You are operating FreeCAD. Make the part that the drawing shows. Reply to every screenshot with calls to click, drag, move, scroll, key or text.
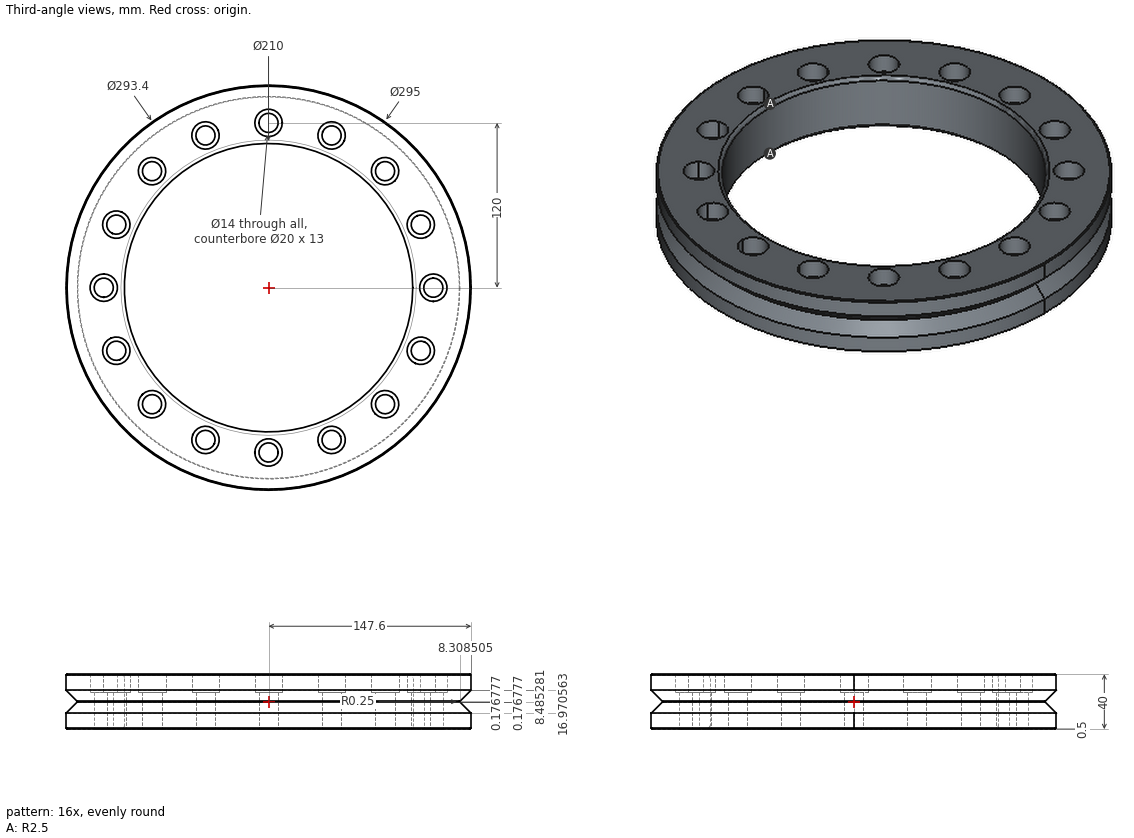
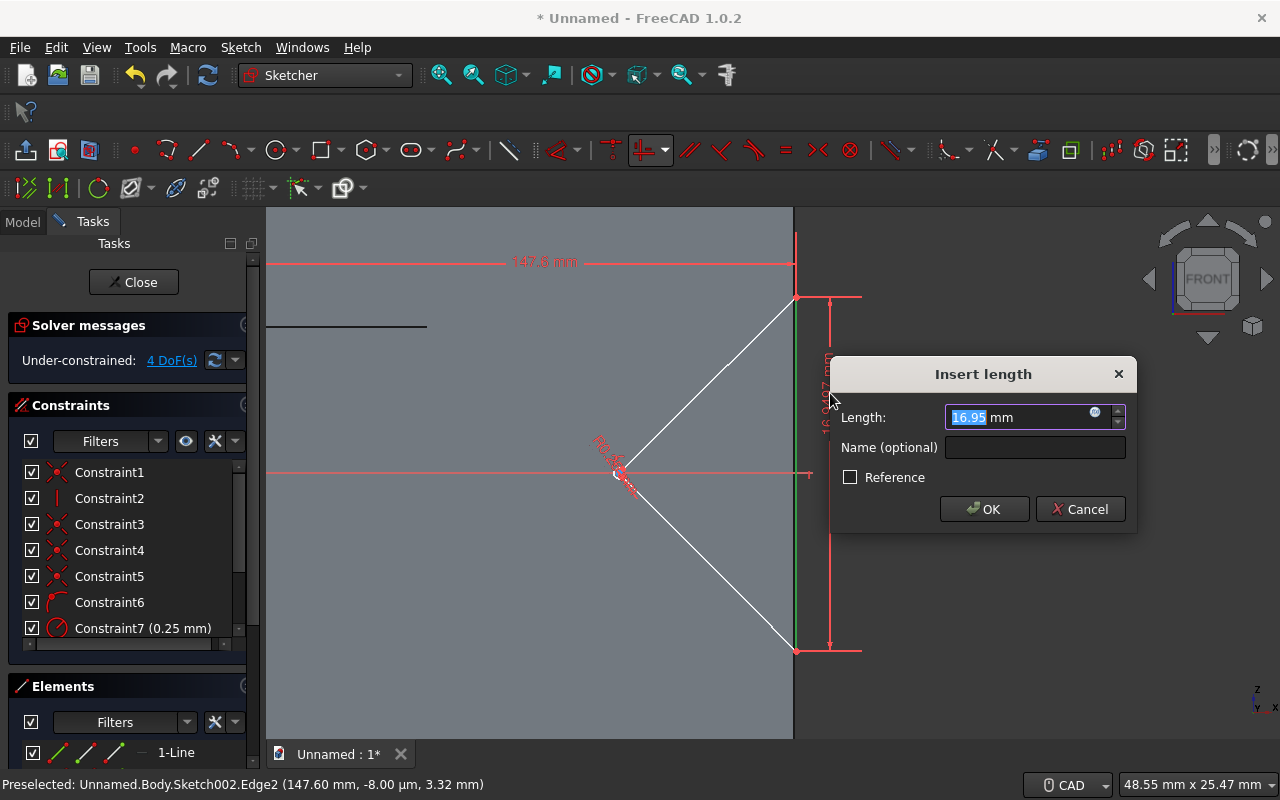
text(16.970563)
key(Return)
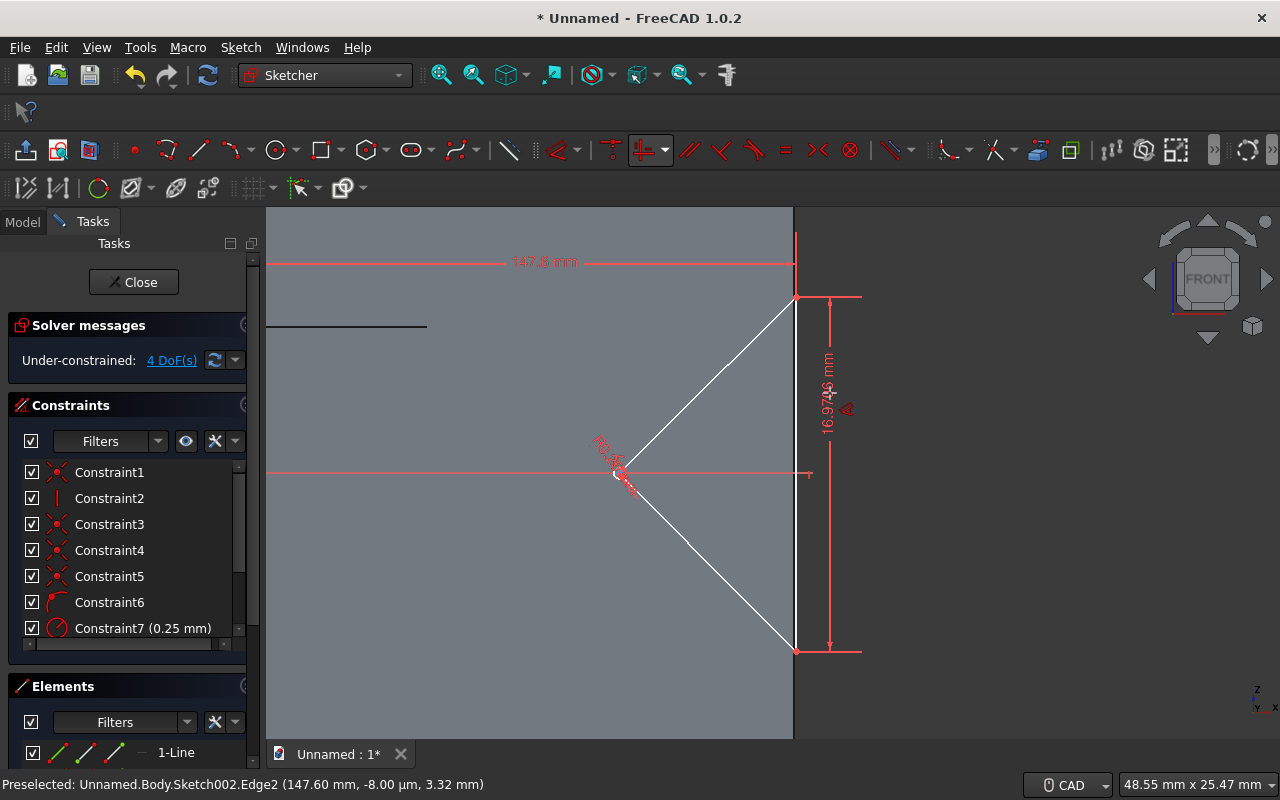
scroll(623, 470, up, 12)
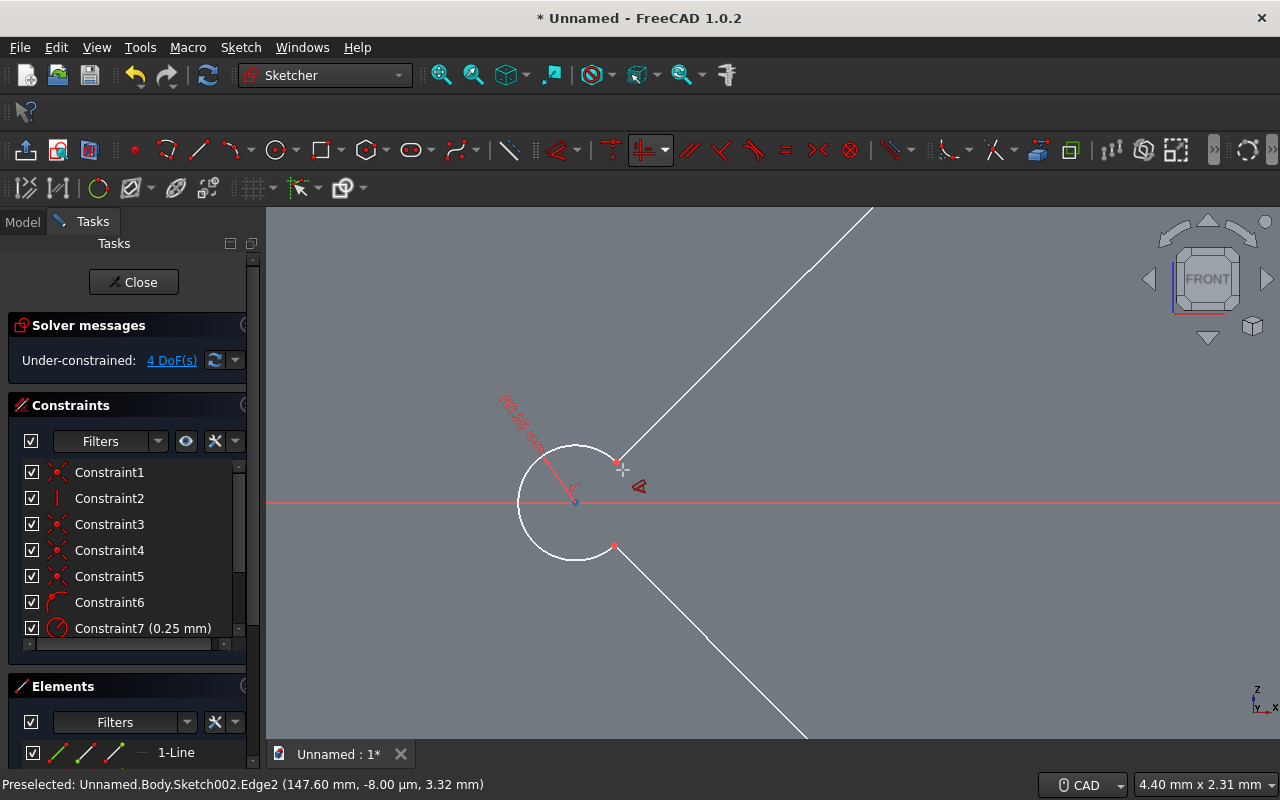
click(617, 462)
click(651, 483)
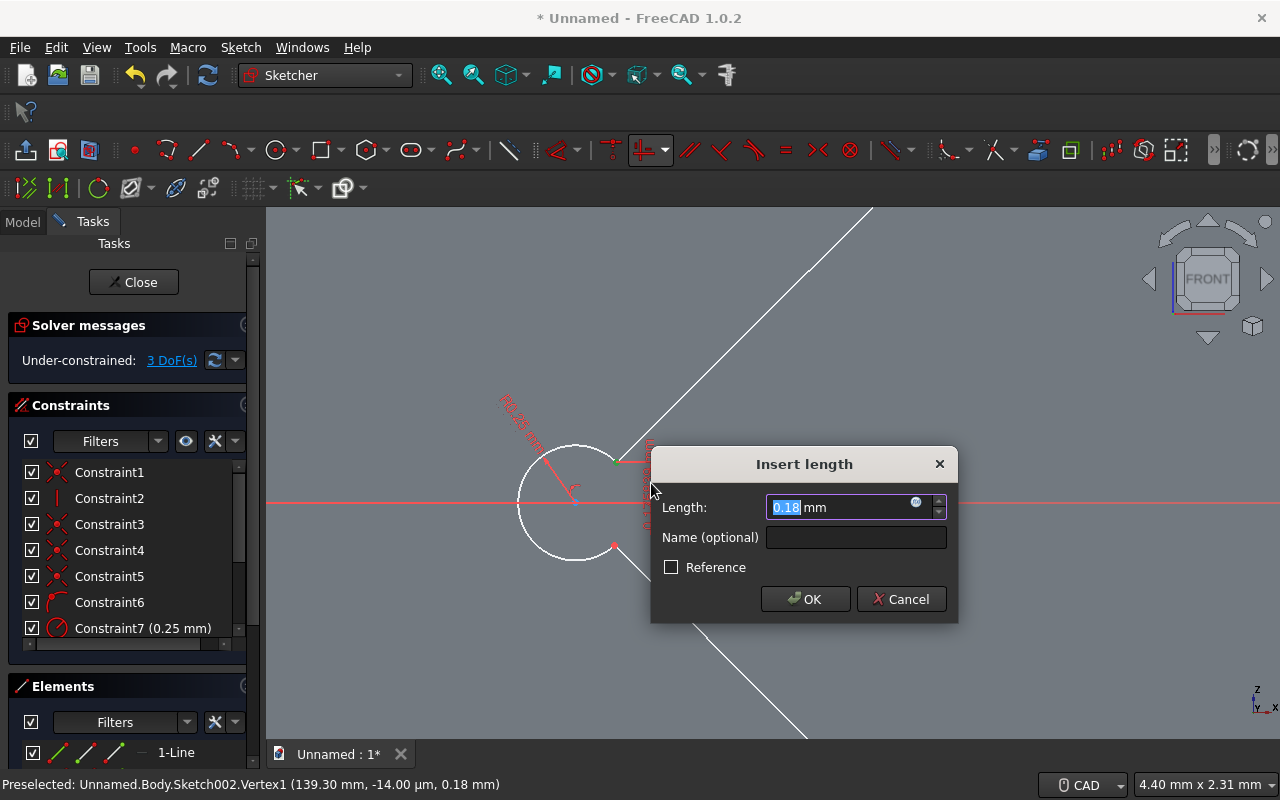
text(0.176777)
key(Return)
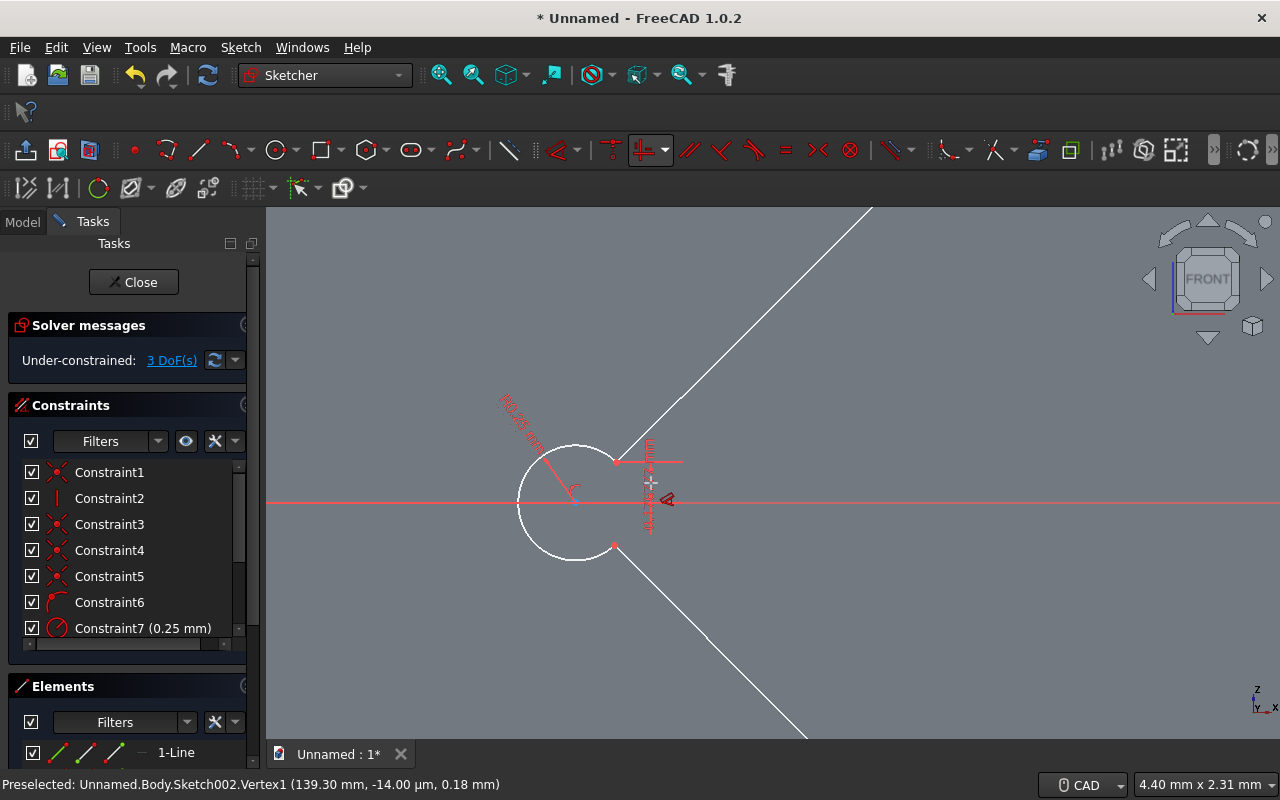
scroll(623, 470, down, 12)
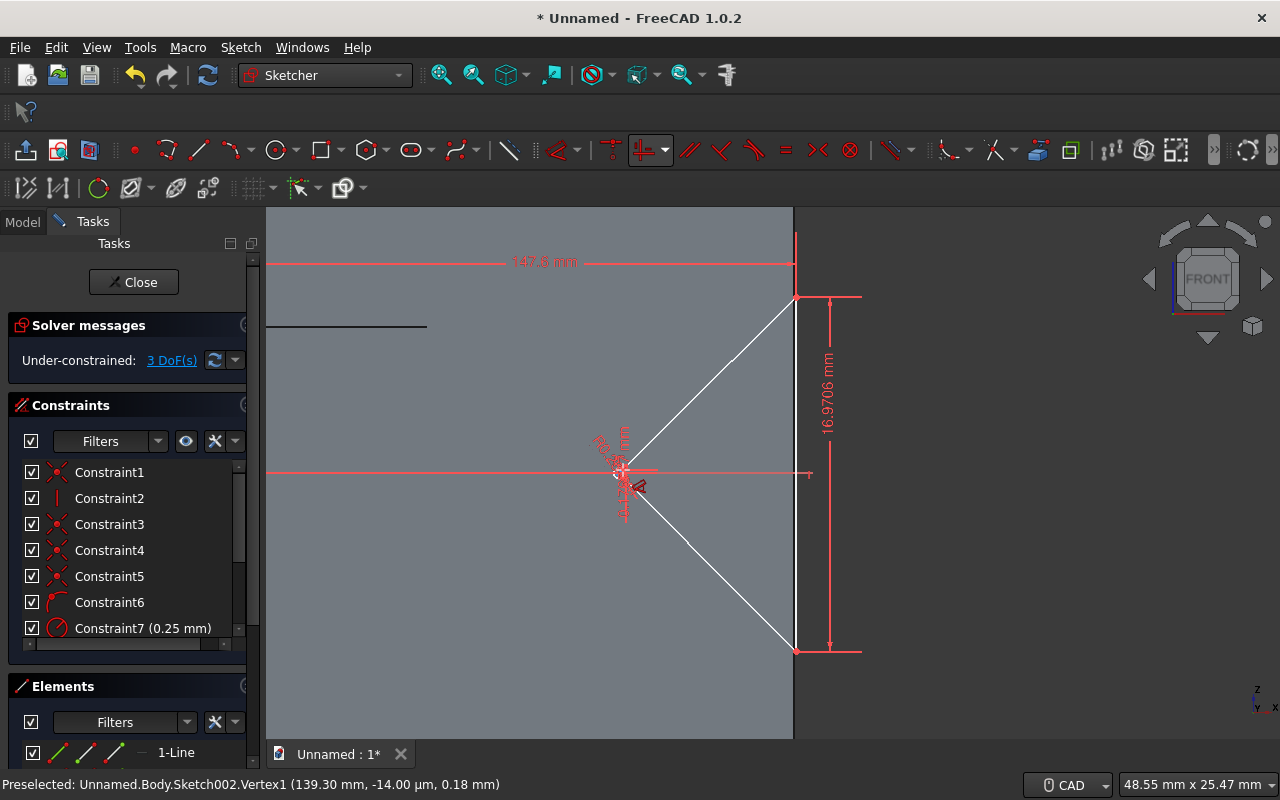
click(796, 297)
click(830, 345)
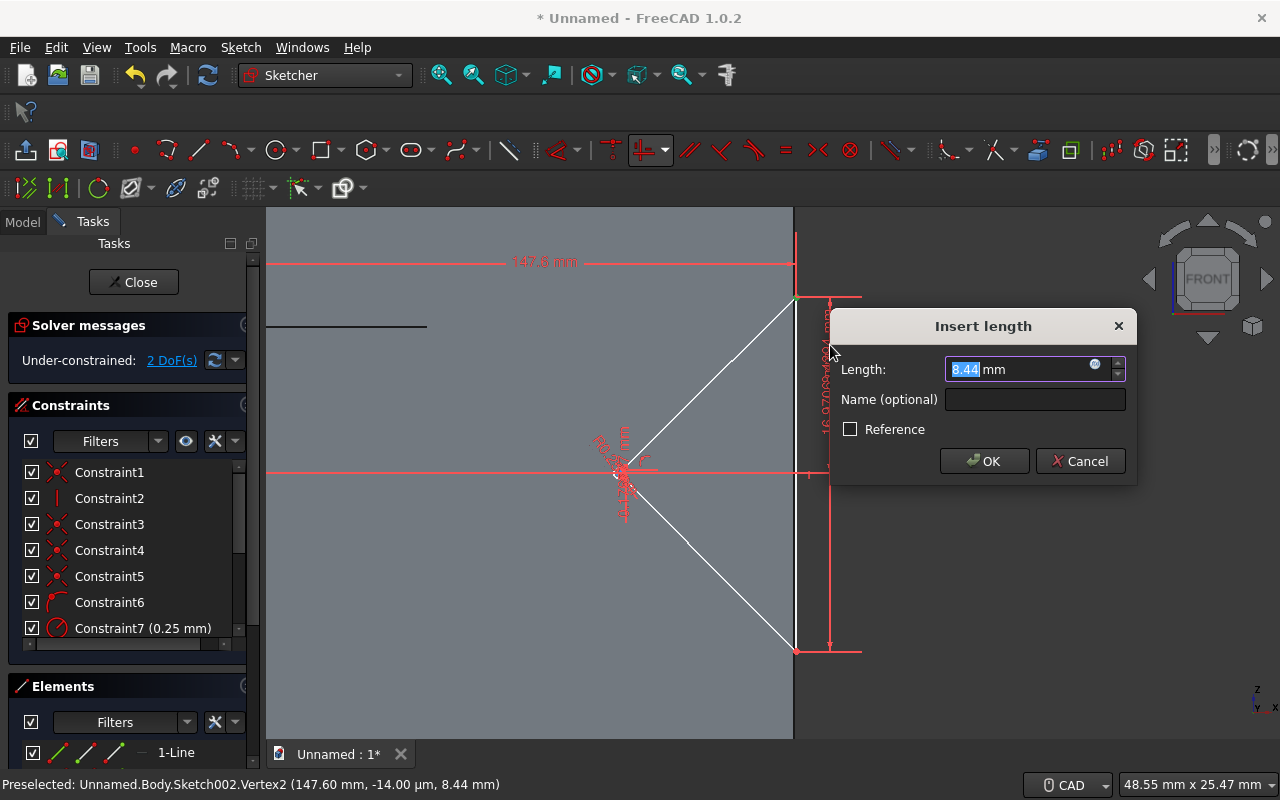
text(8.485281)
key(Return)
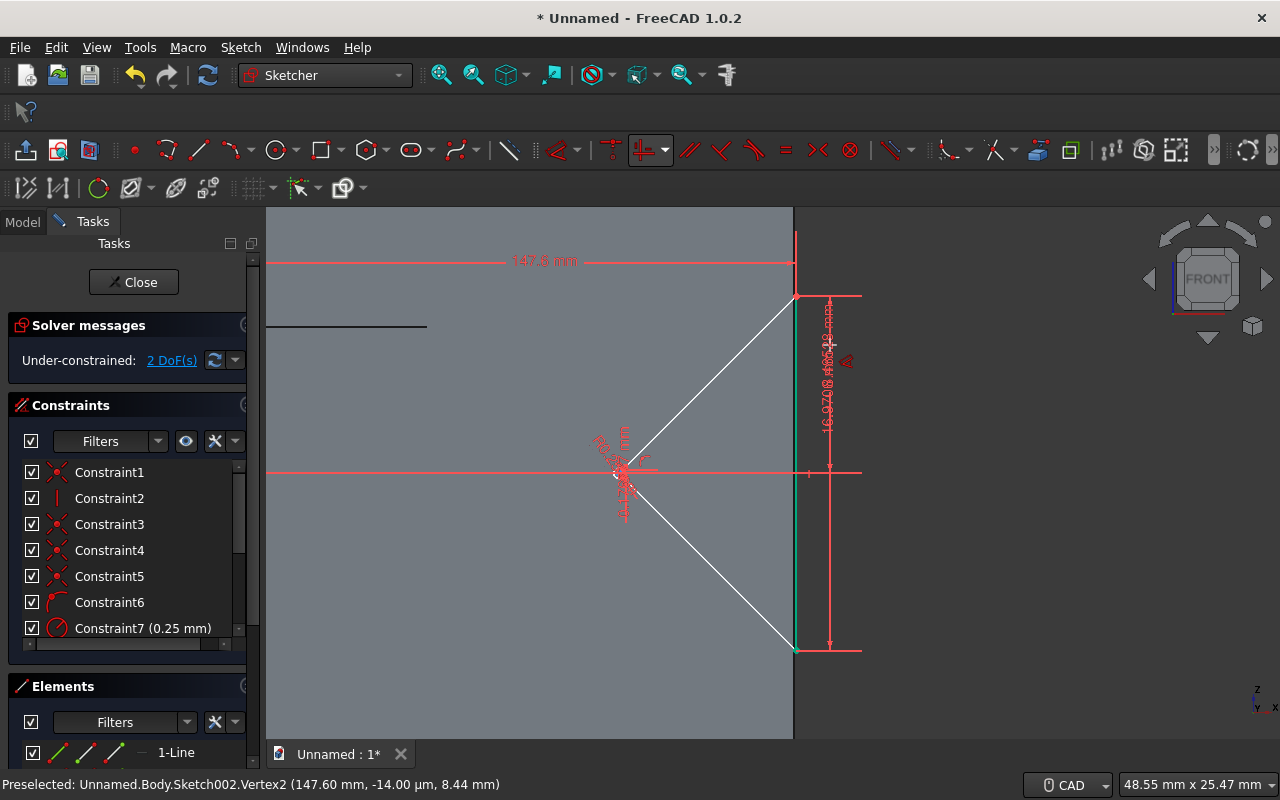
scroll(623, 477, up, 12)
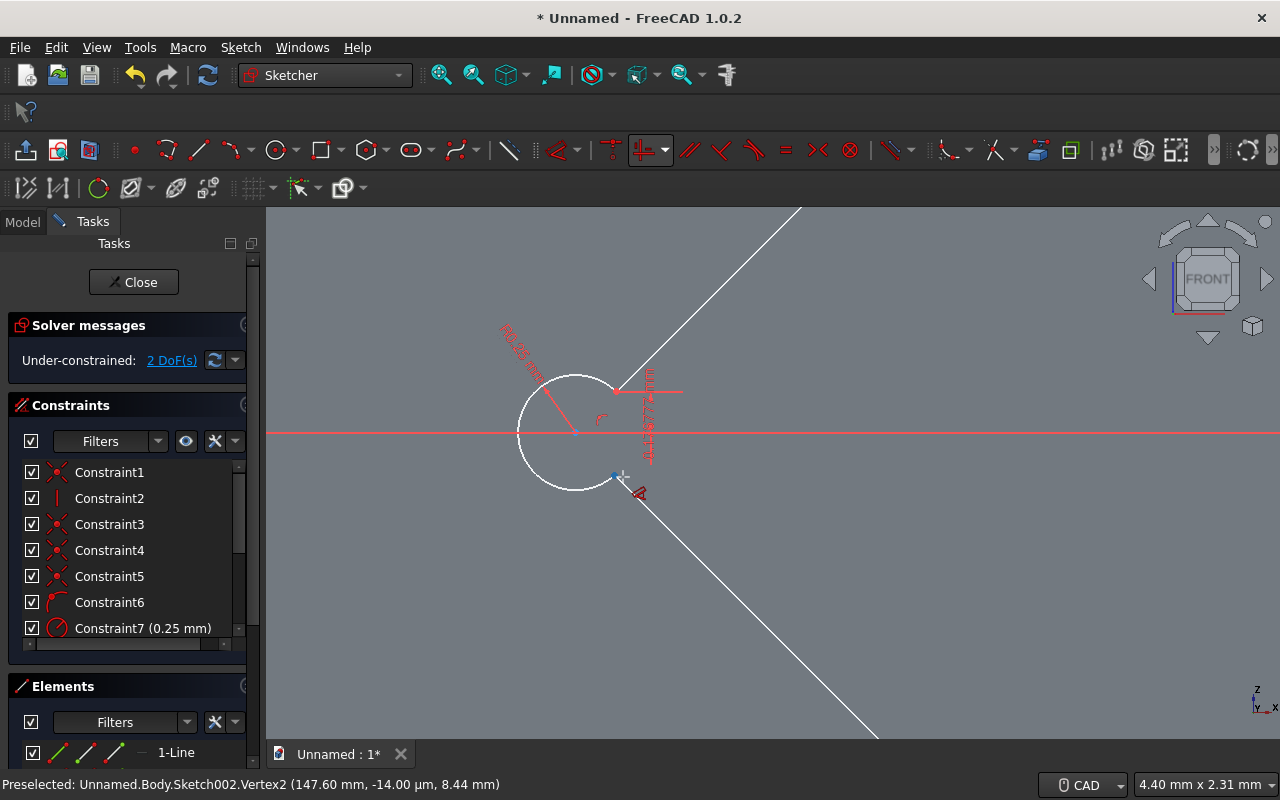
click(615, 475)
click(649, 454)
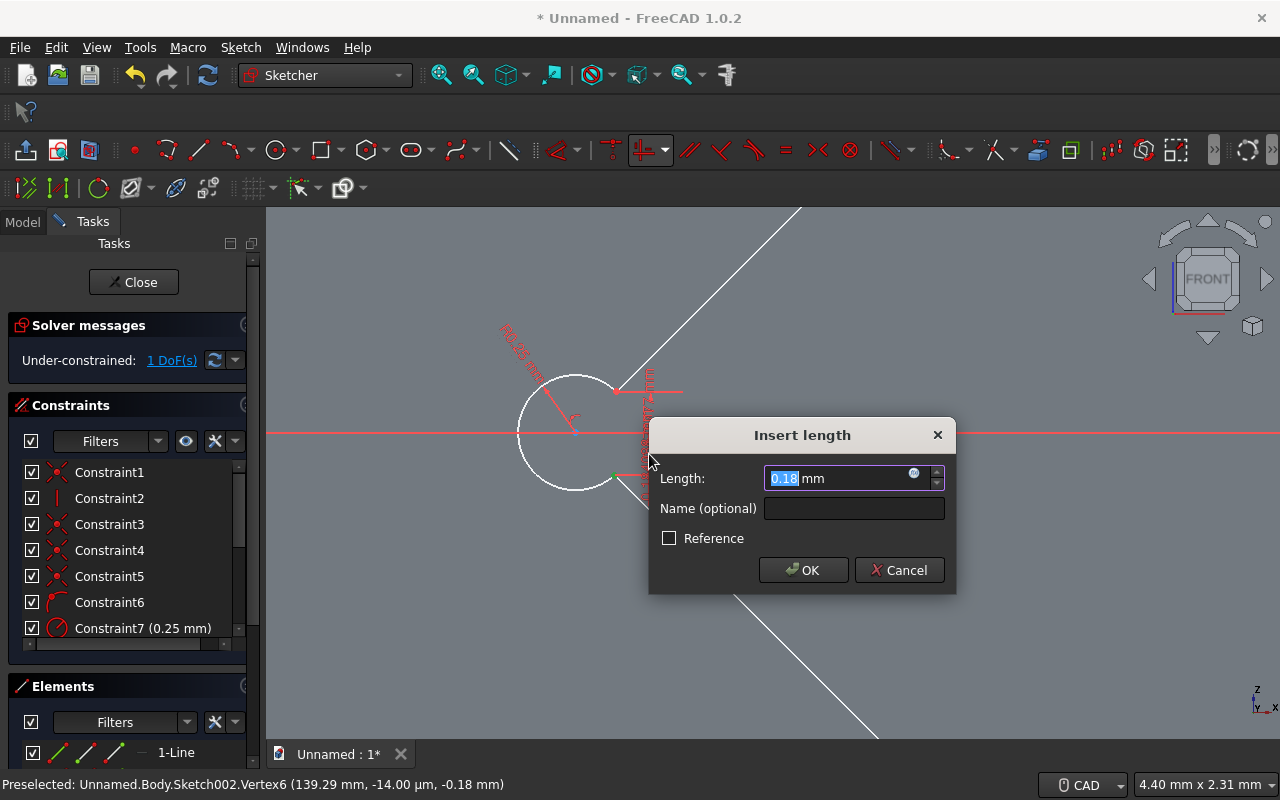
text(0.176777)
key(Return)